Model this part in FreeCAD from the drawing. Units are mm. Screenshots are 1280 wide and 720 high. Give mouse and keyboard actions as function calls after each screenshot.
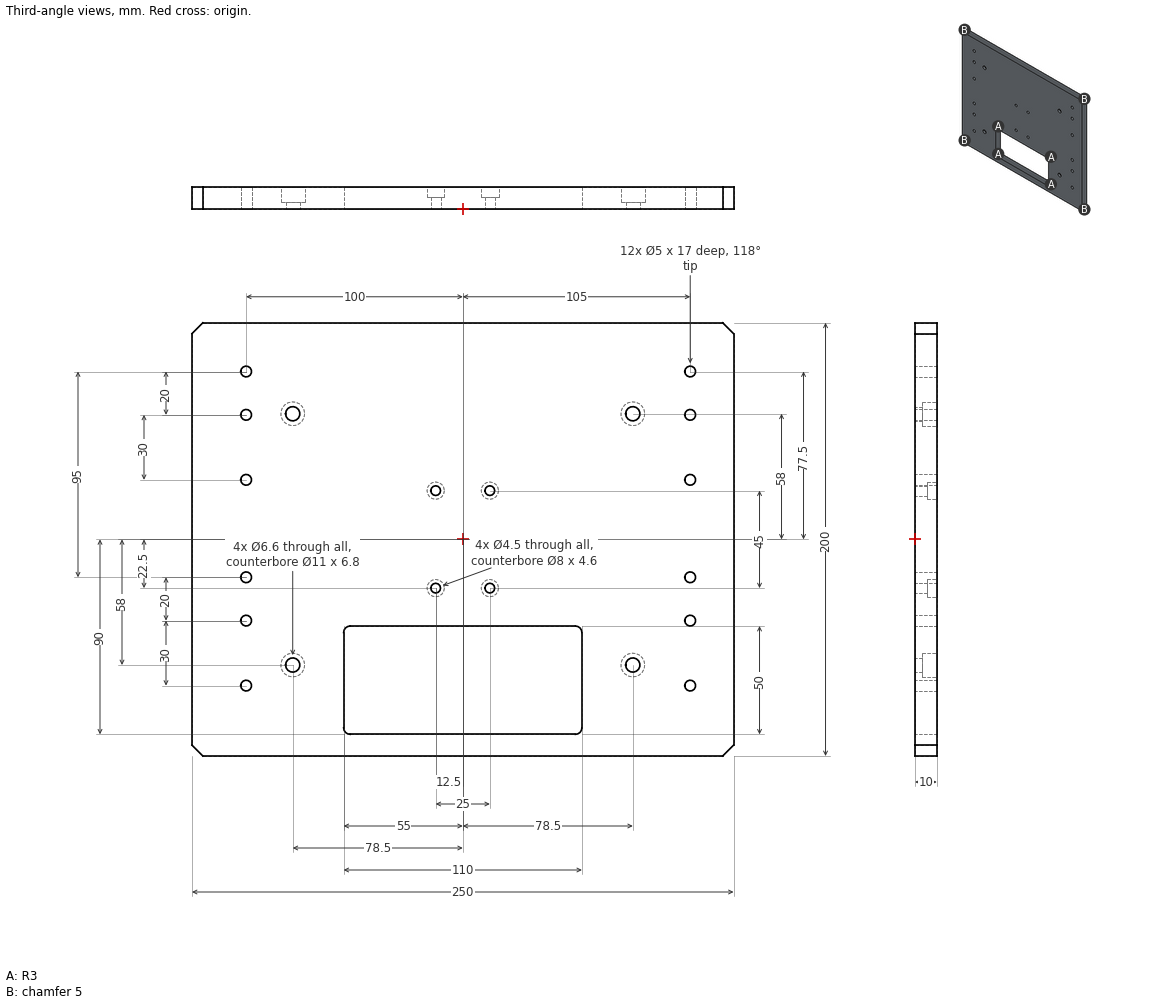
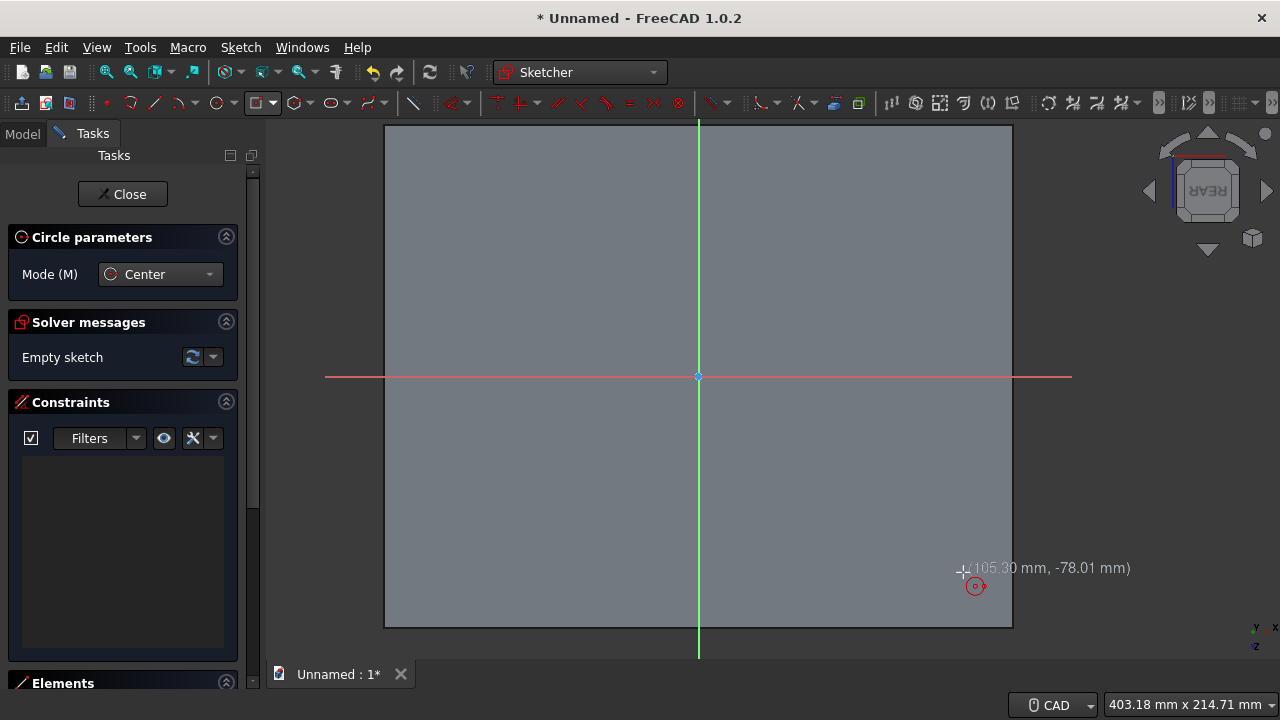
click(963, 572)
move(967, 567)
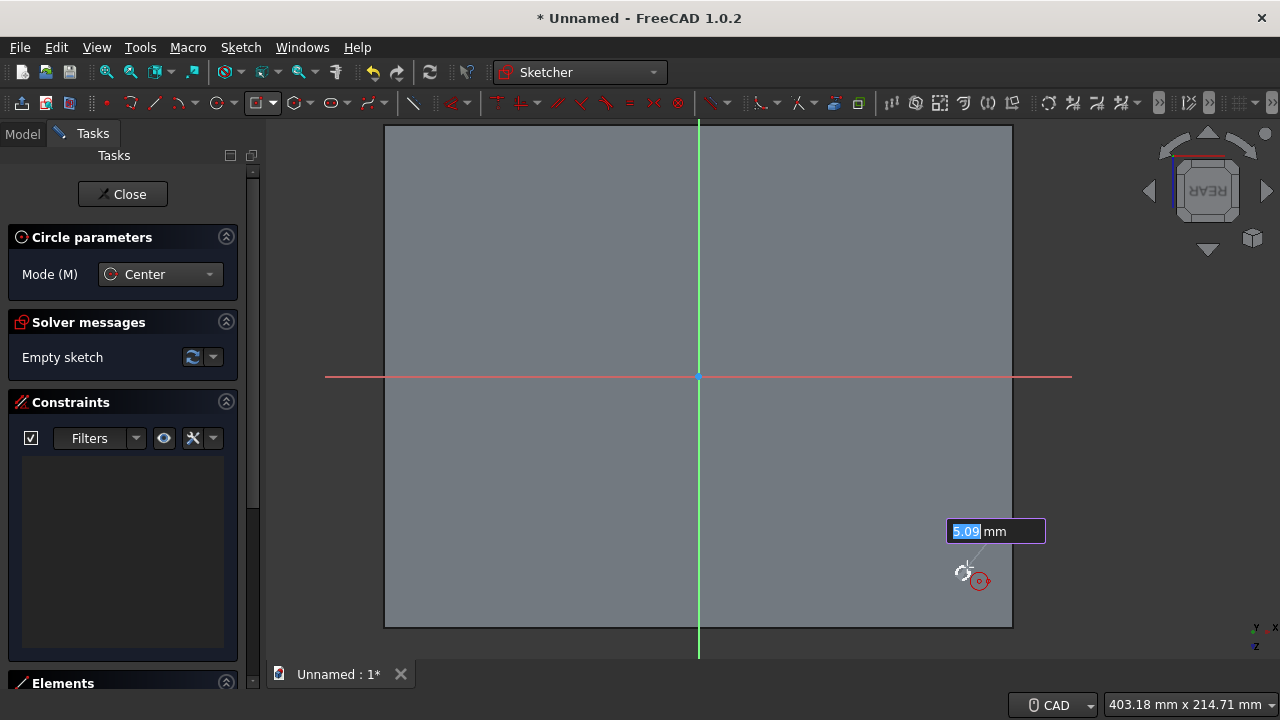
text(5)
key(Return)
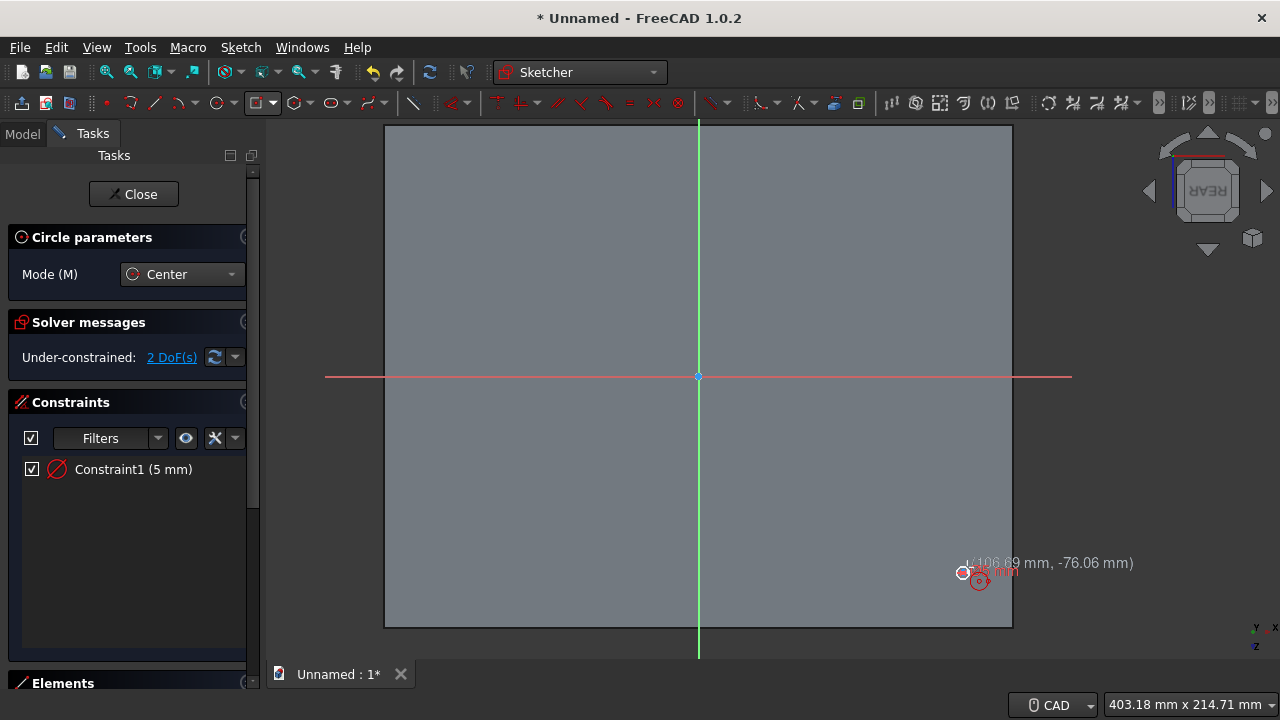
scroll(447, 572, up, 7)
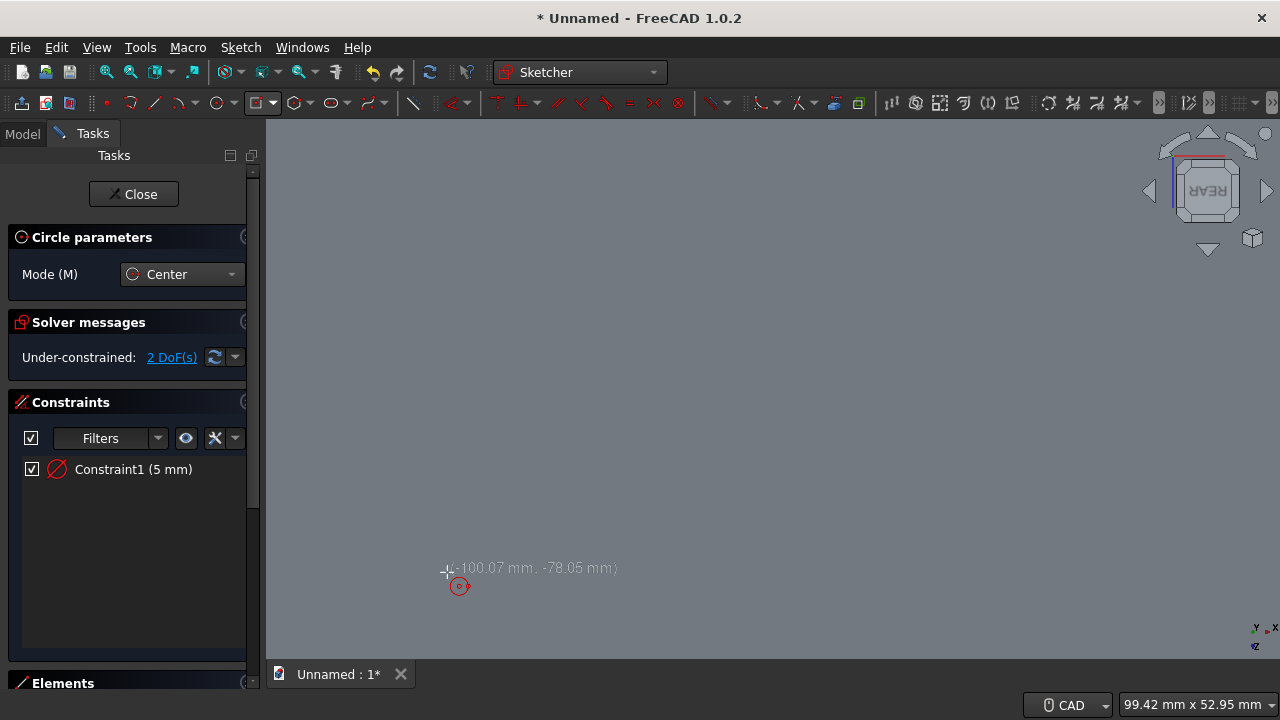
scroll(447, 572, down, 7)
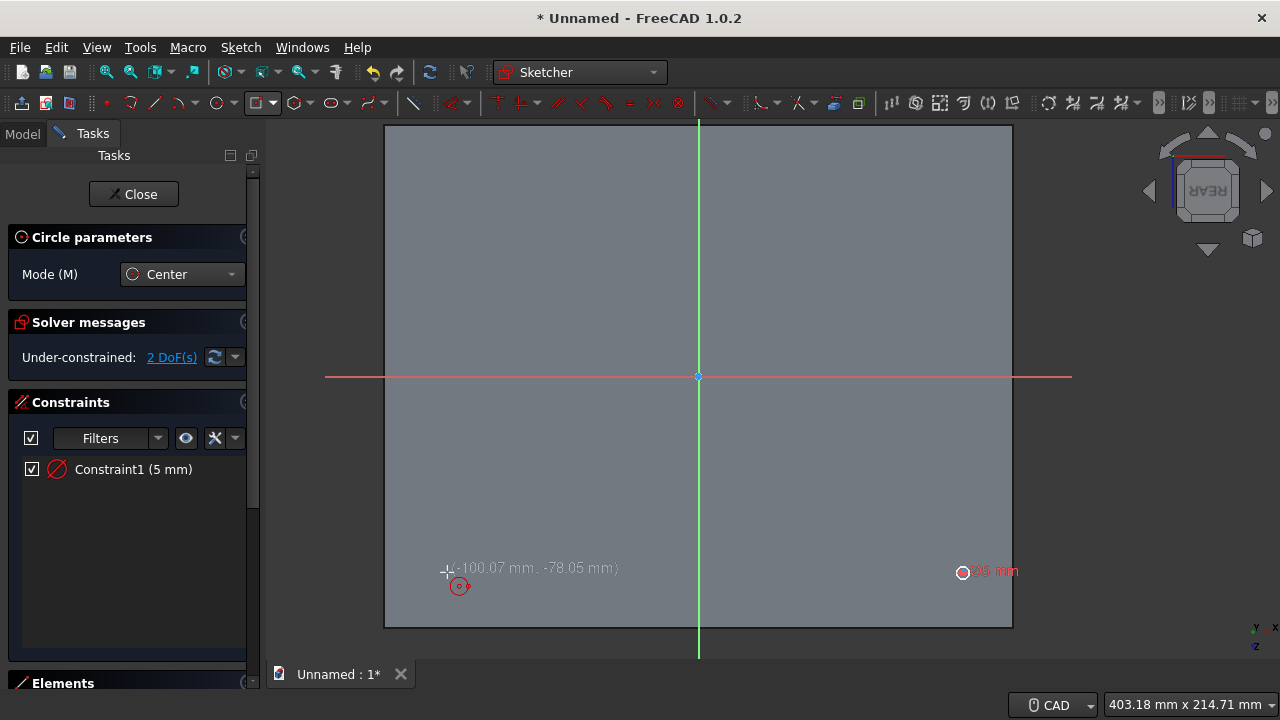
click(447, 572)
move(452, 567)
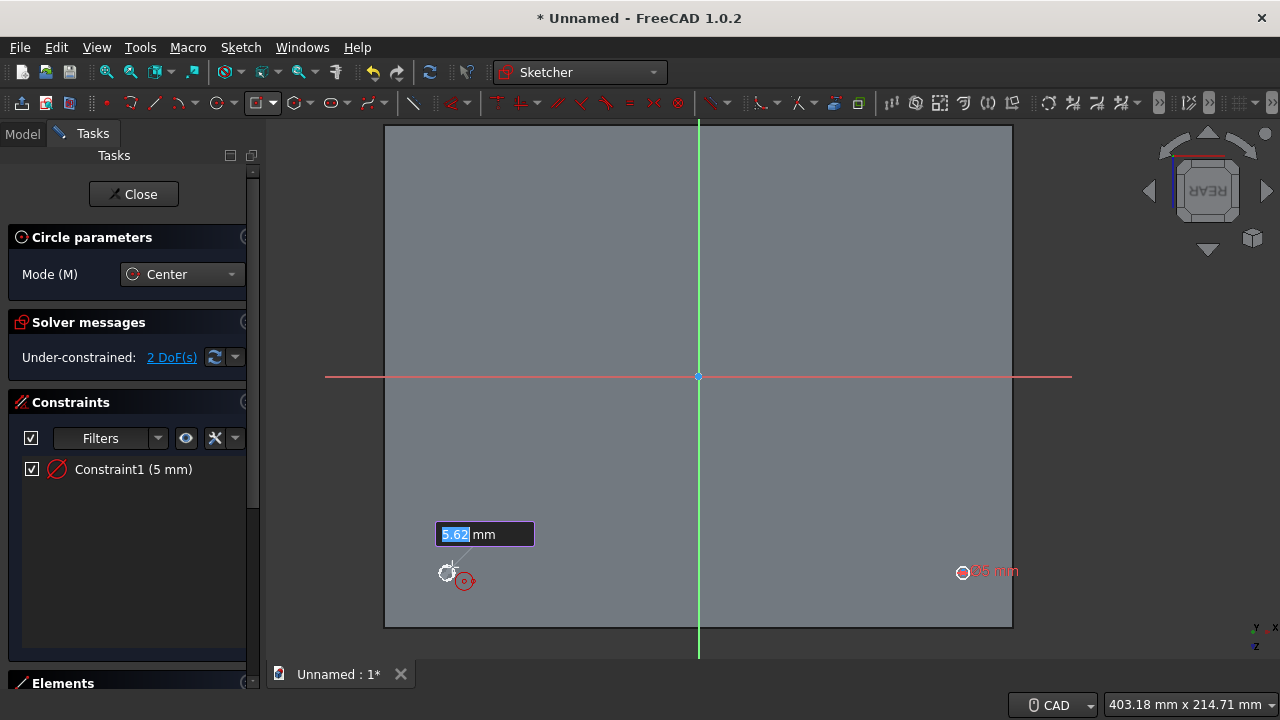
text(5)
key(Return)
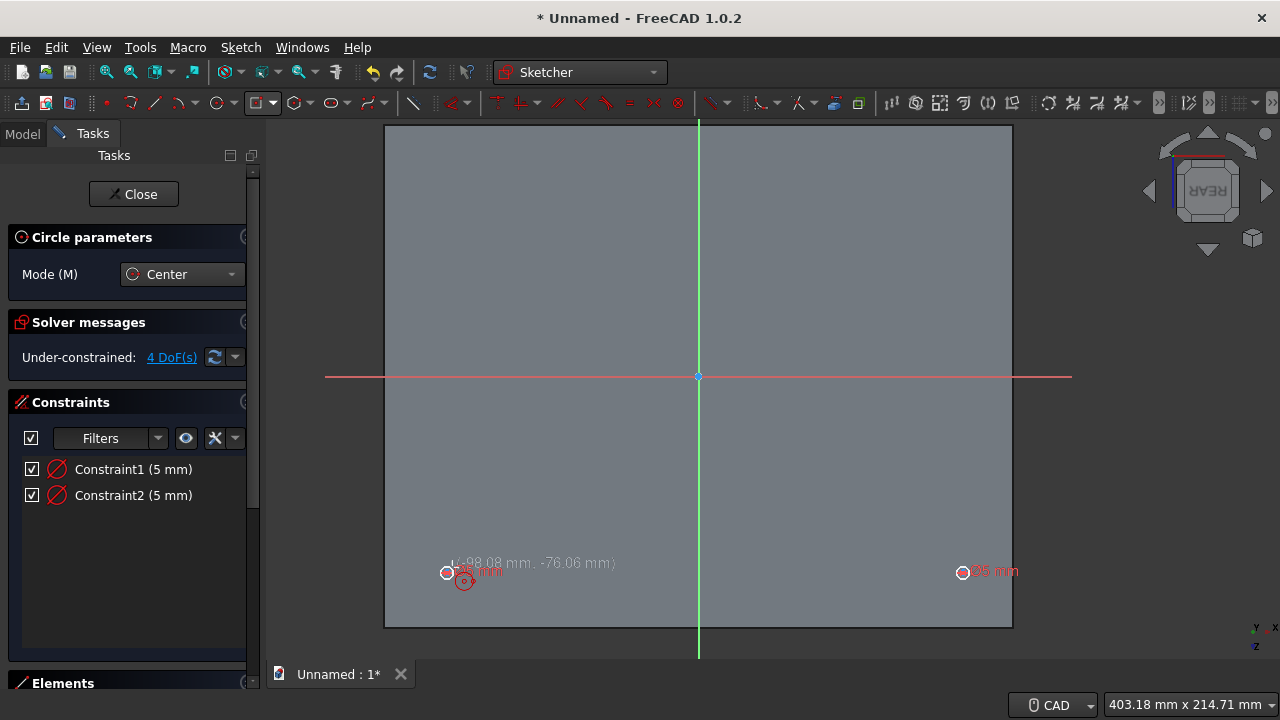
scroll(447, 333, up, 7)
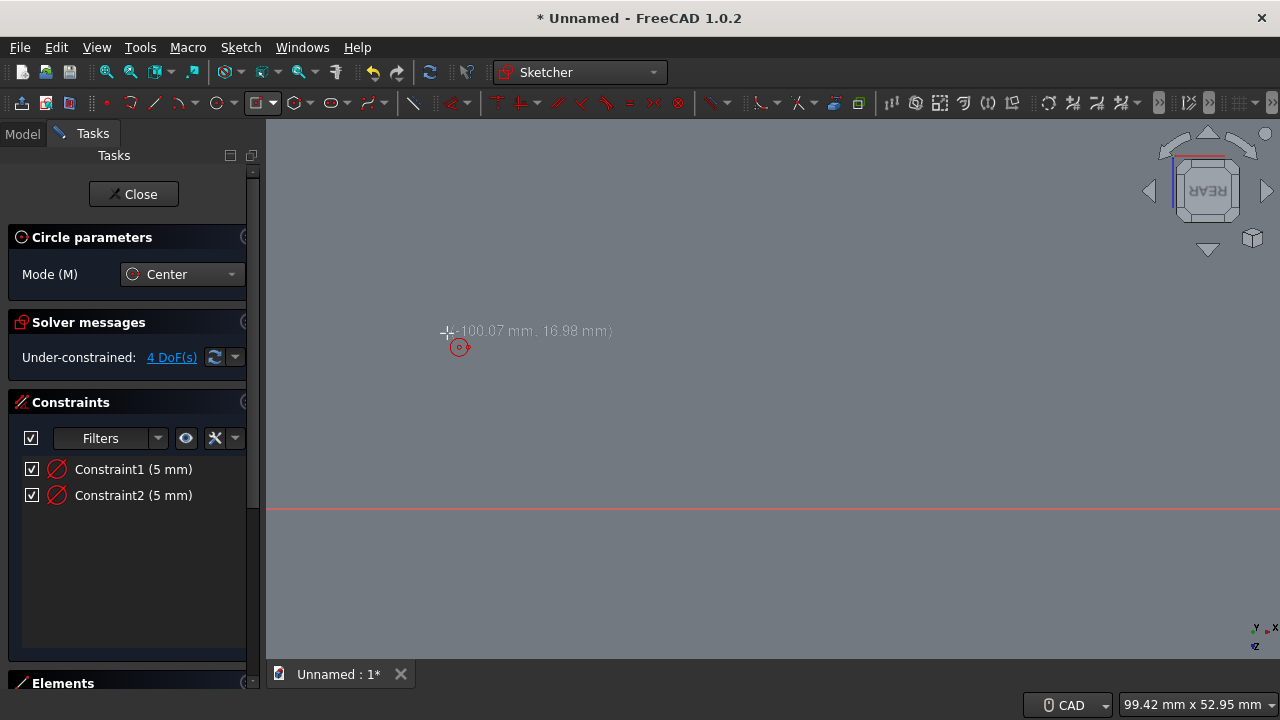
scroll(447, 333, down, 7)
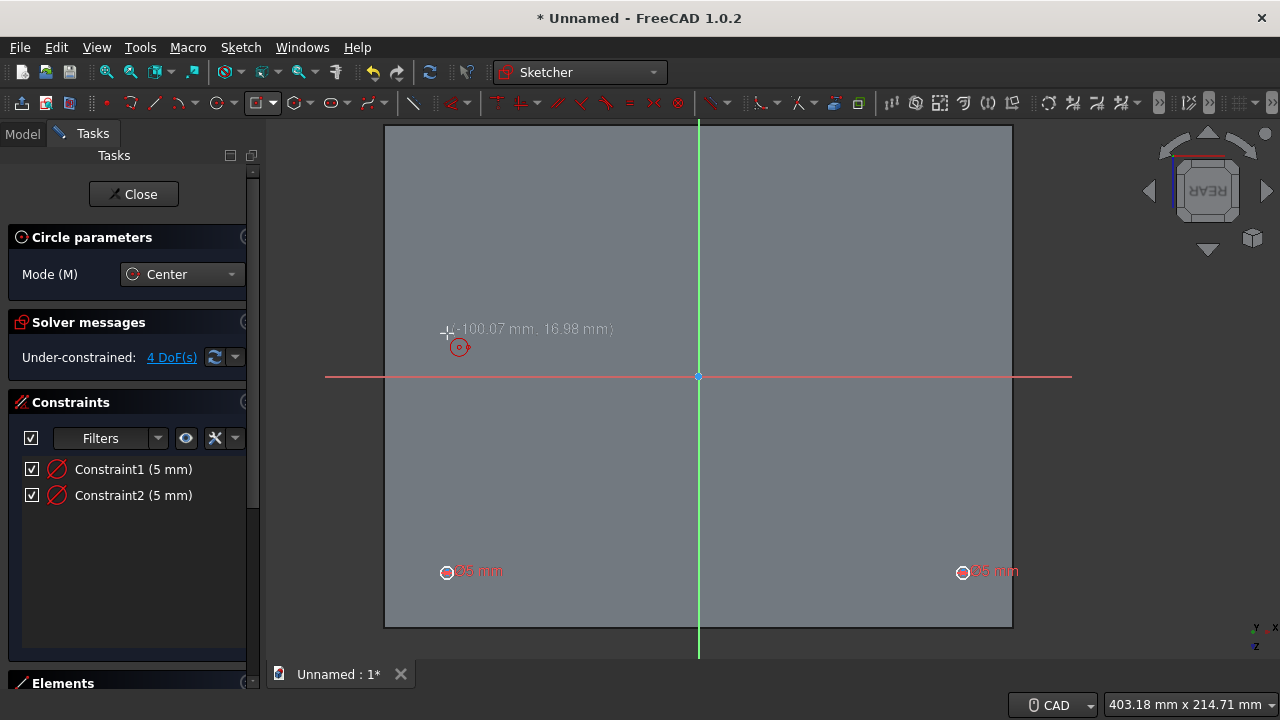
click(447, 333)
move(452, 328)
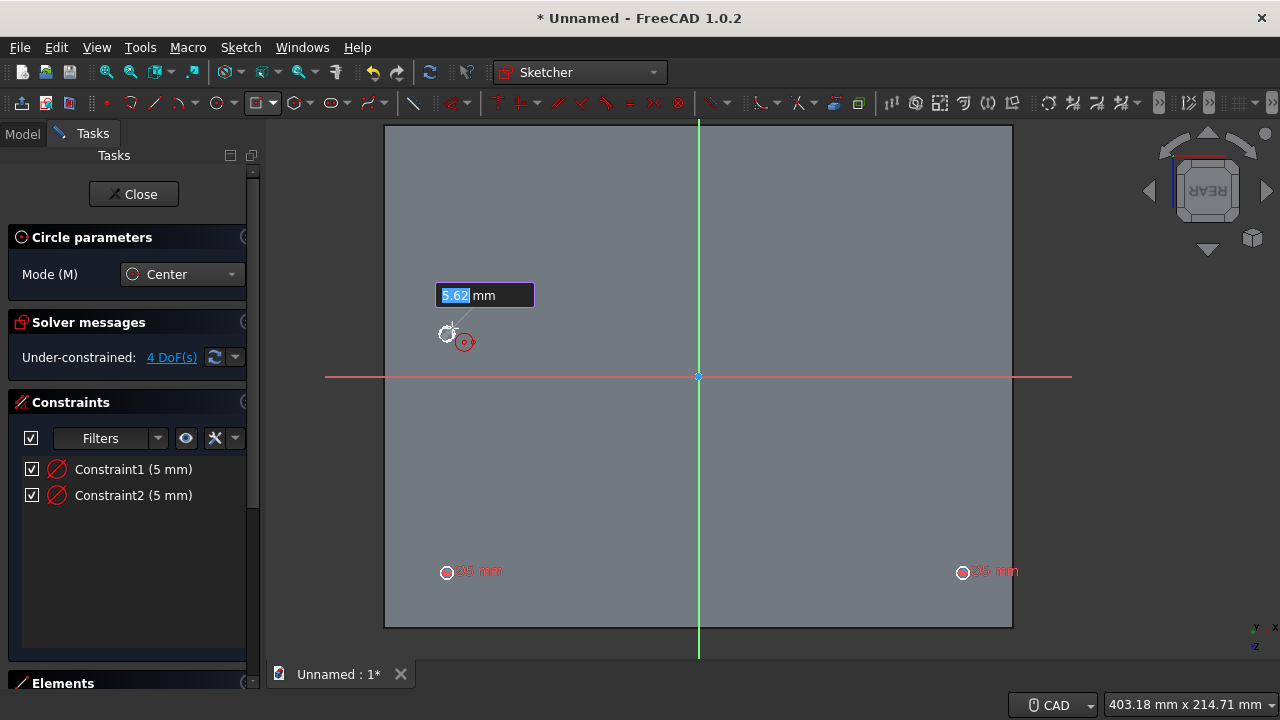
text(5)
key(Return)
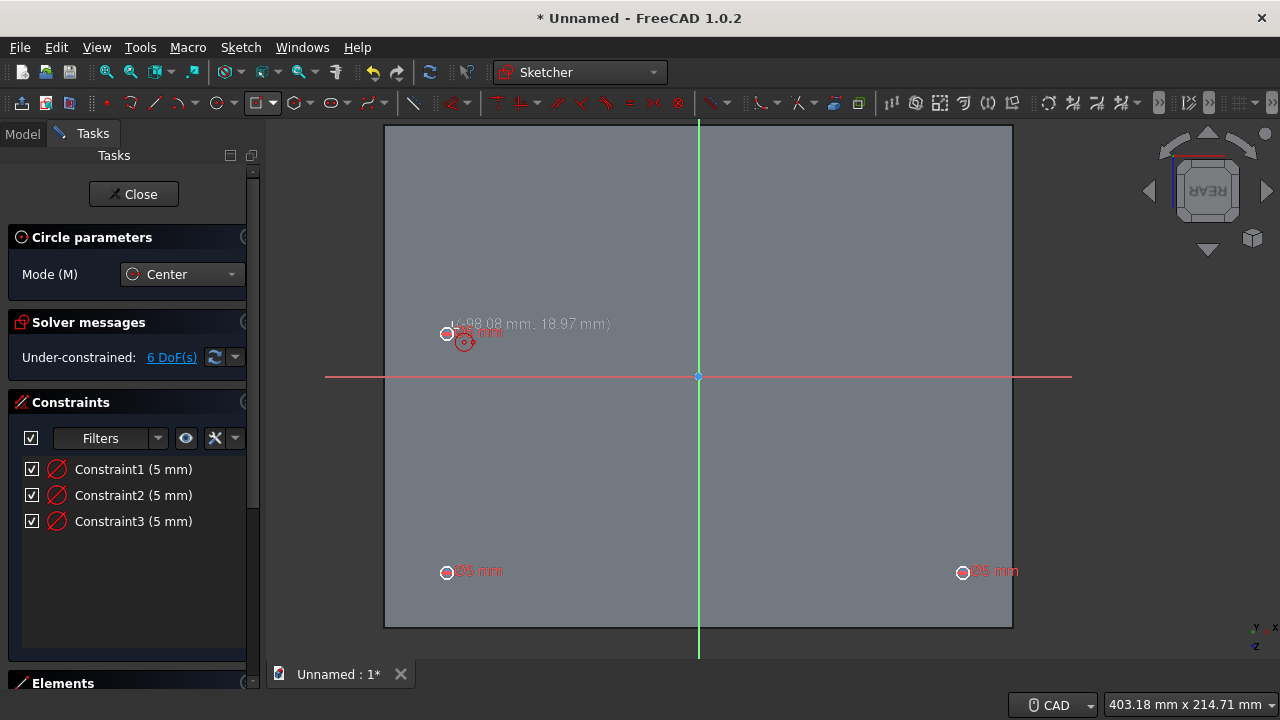
scroll(963, 333, up, 7)